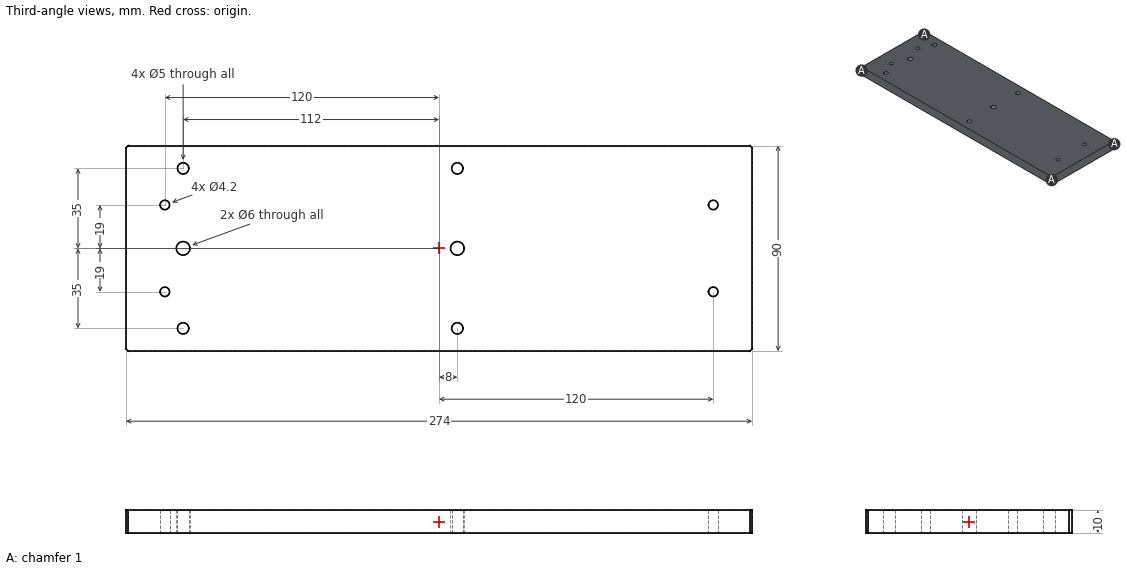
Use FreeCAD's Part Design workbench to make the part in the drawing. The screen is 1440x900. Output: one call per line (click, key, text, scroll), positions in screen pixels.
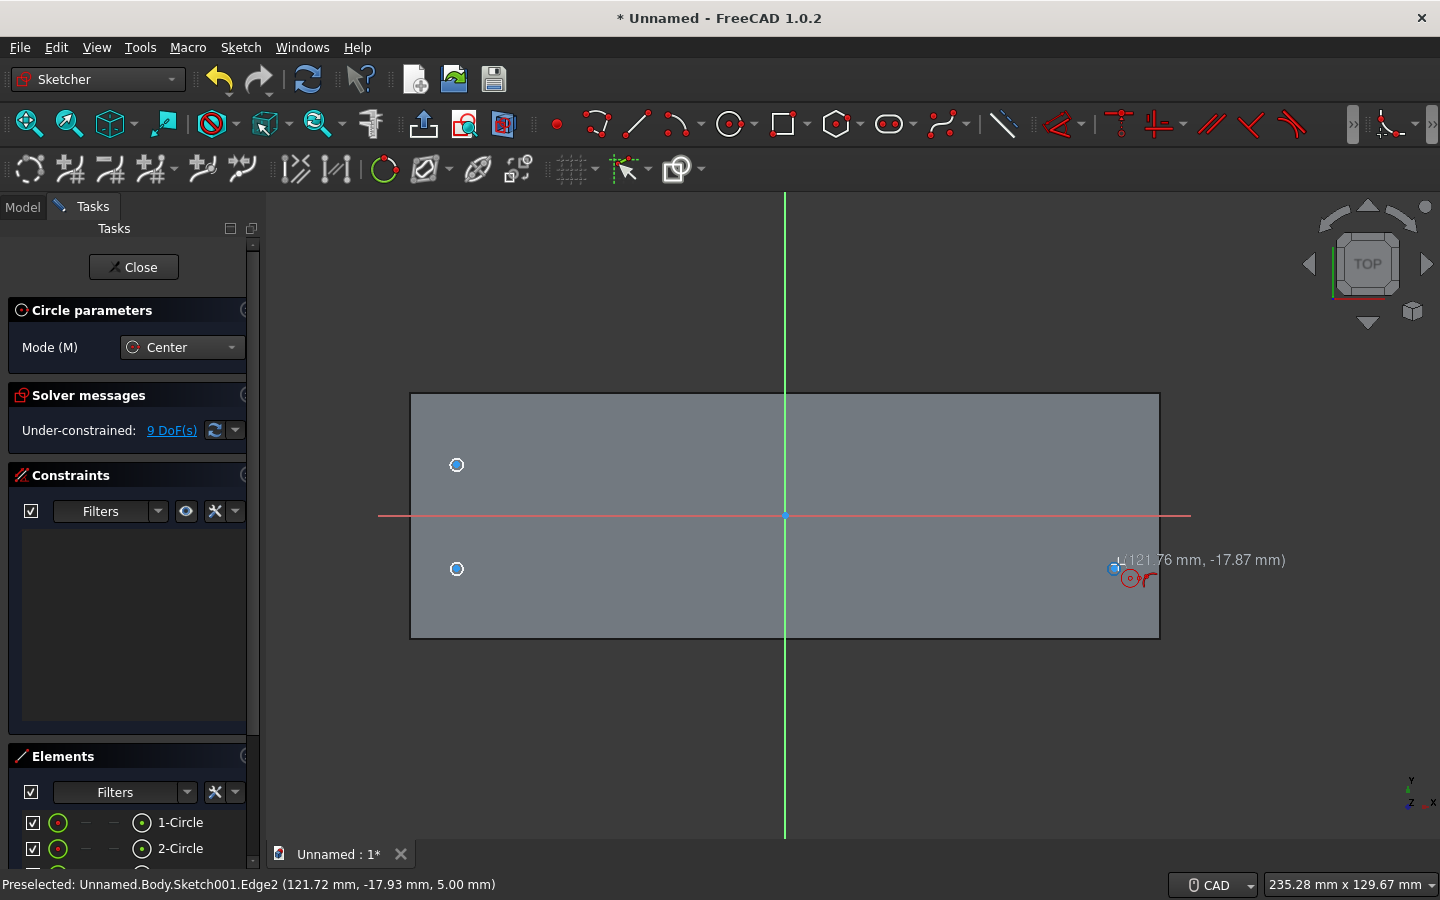
click(1114, 464)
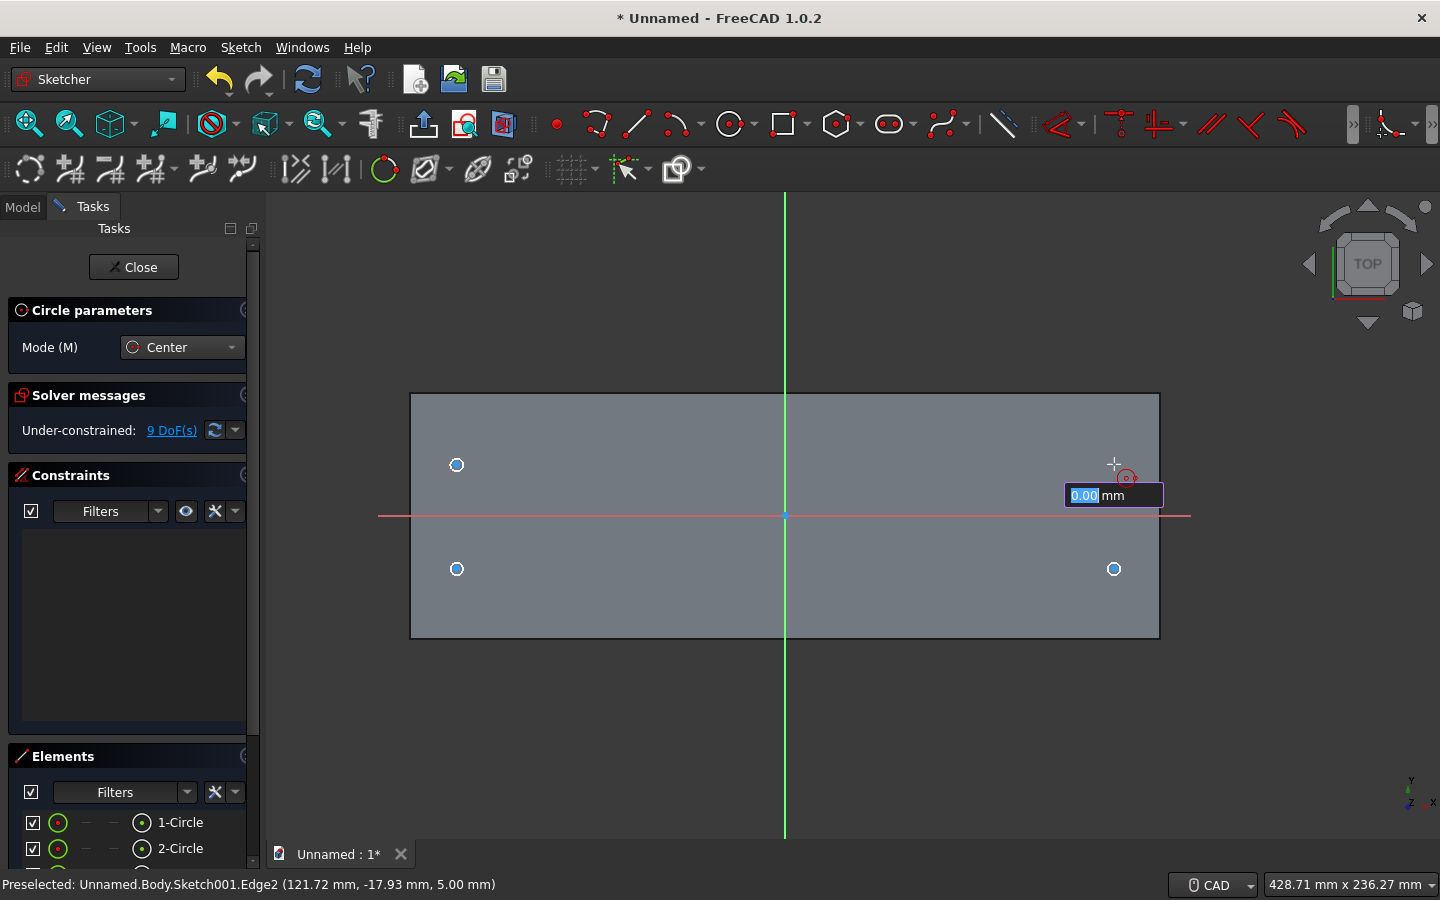
scroll(1118, 460, up, 6)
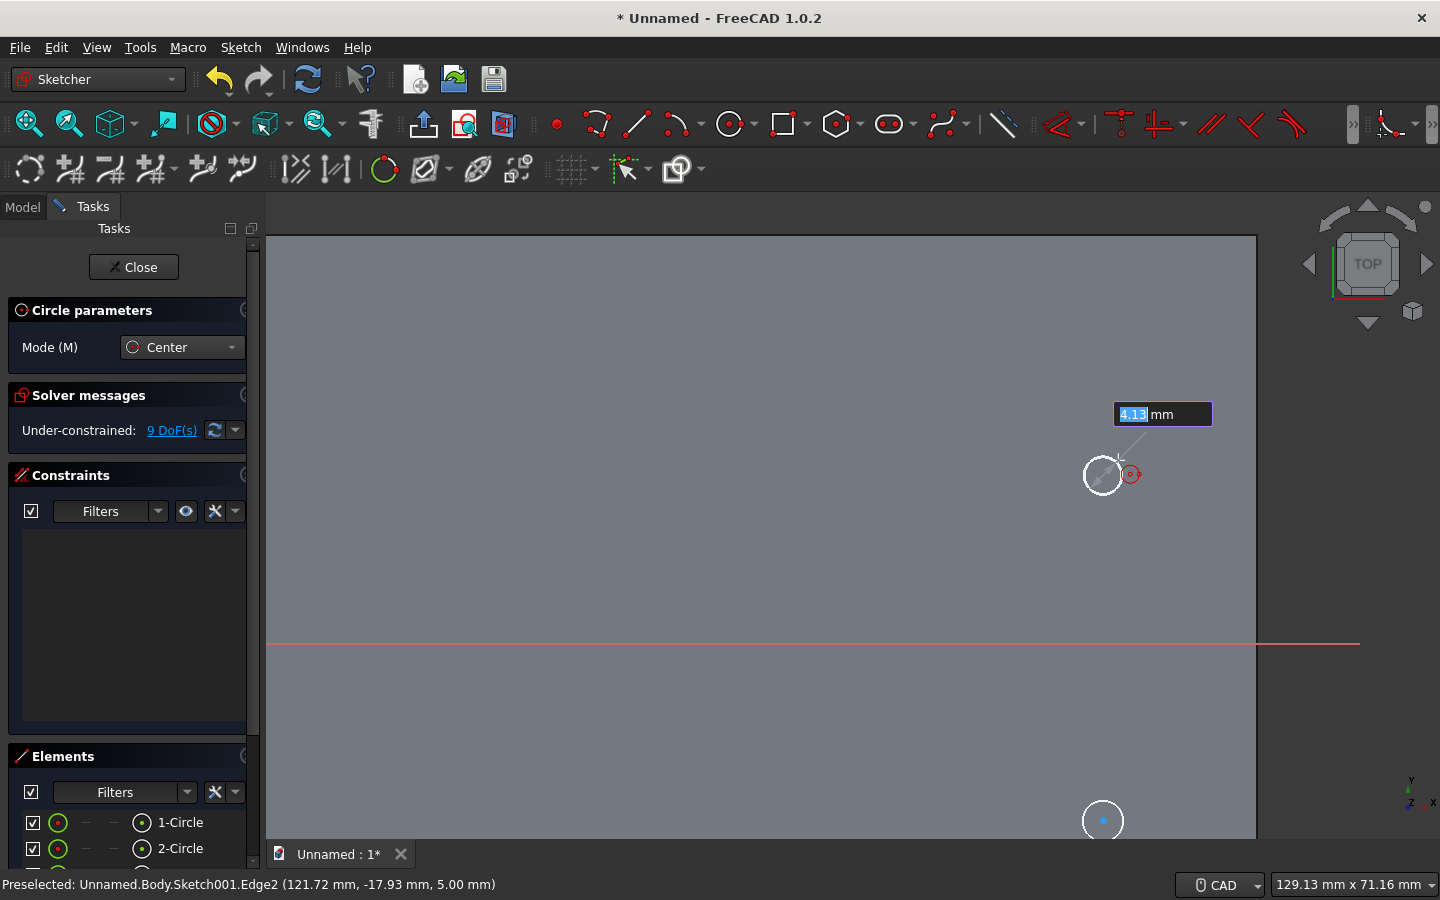
click(1115, 458)
key(Escape)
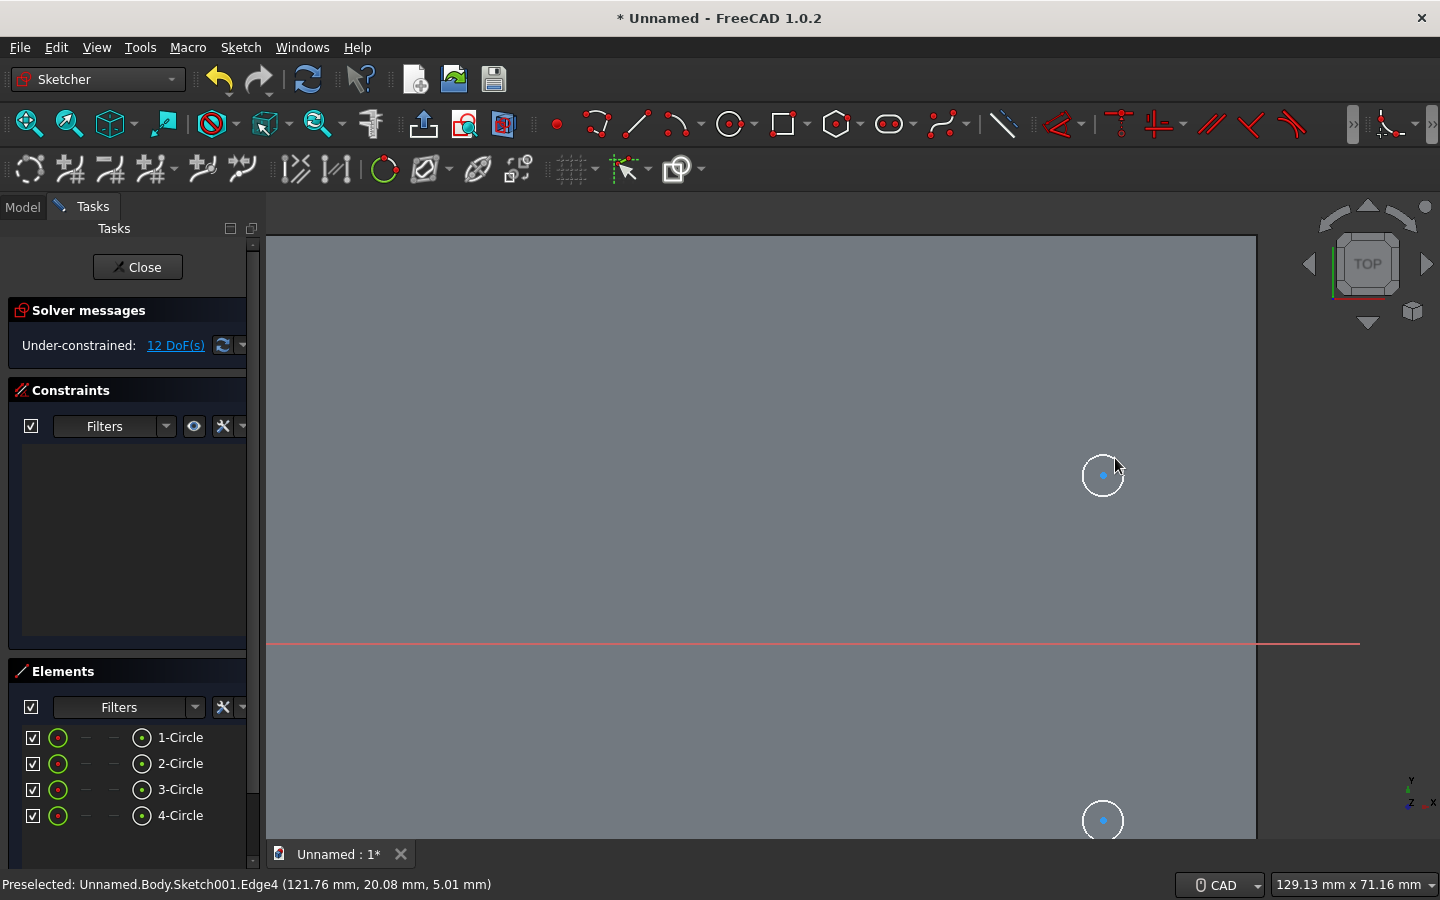
scroll(1118, 460, down, 6)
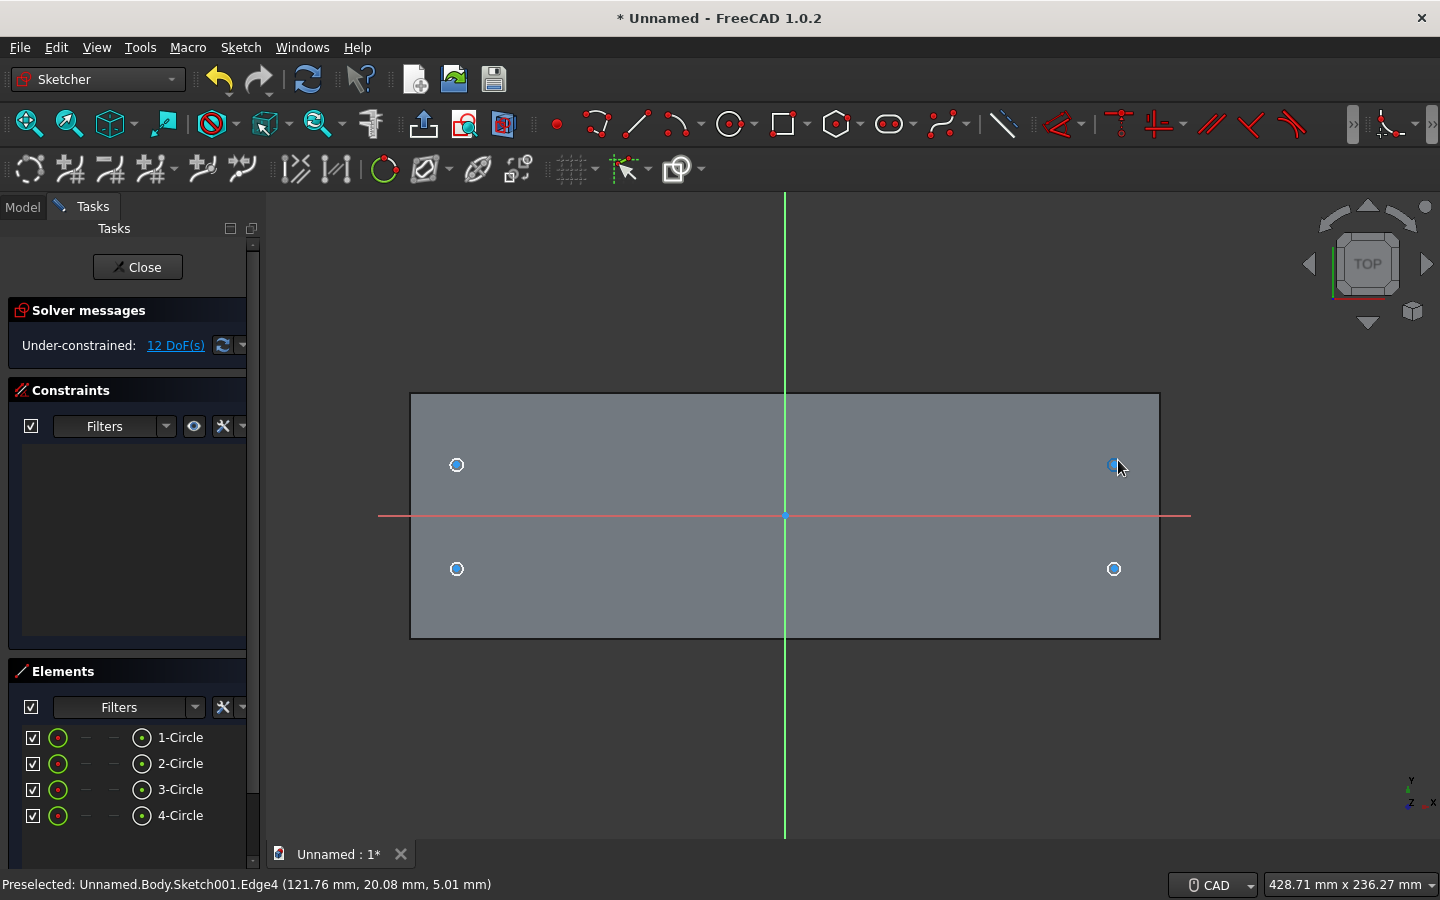
scroll(461, 461, up, 4)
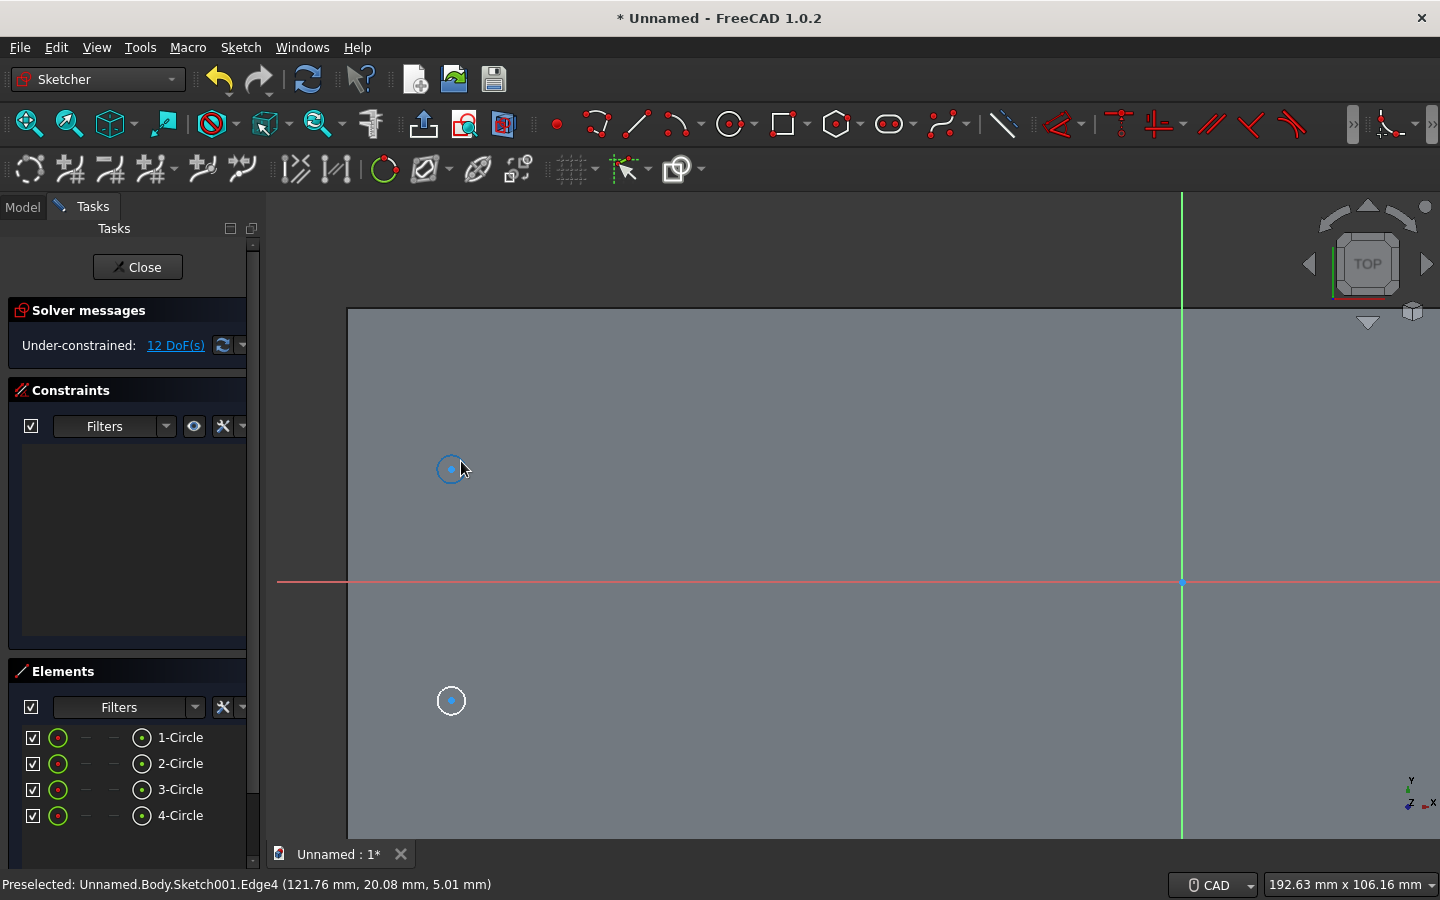
click(461, 459)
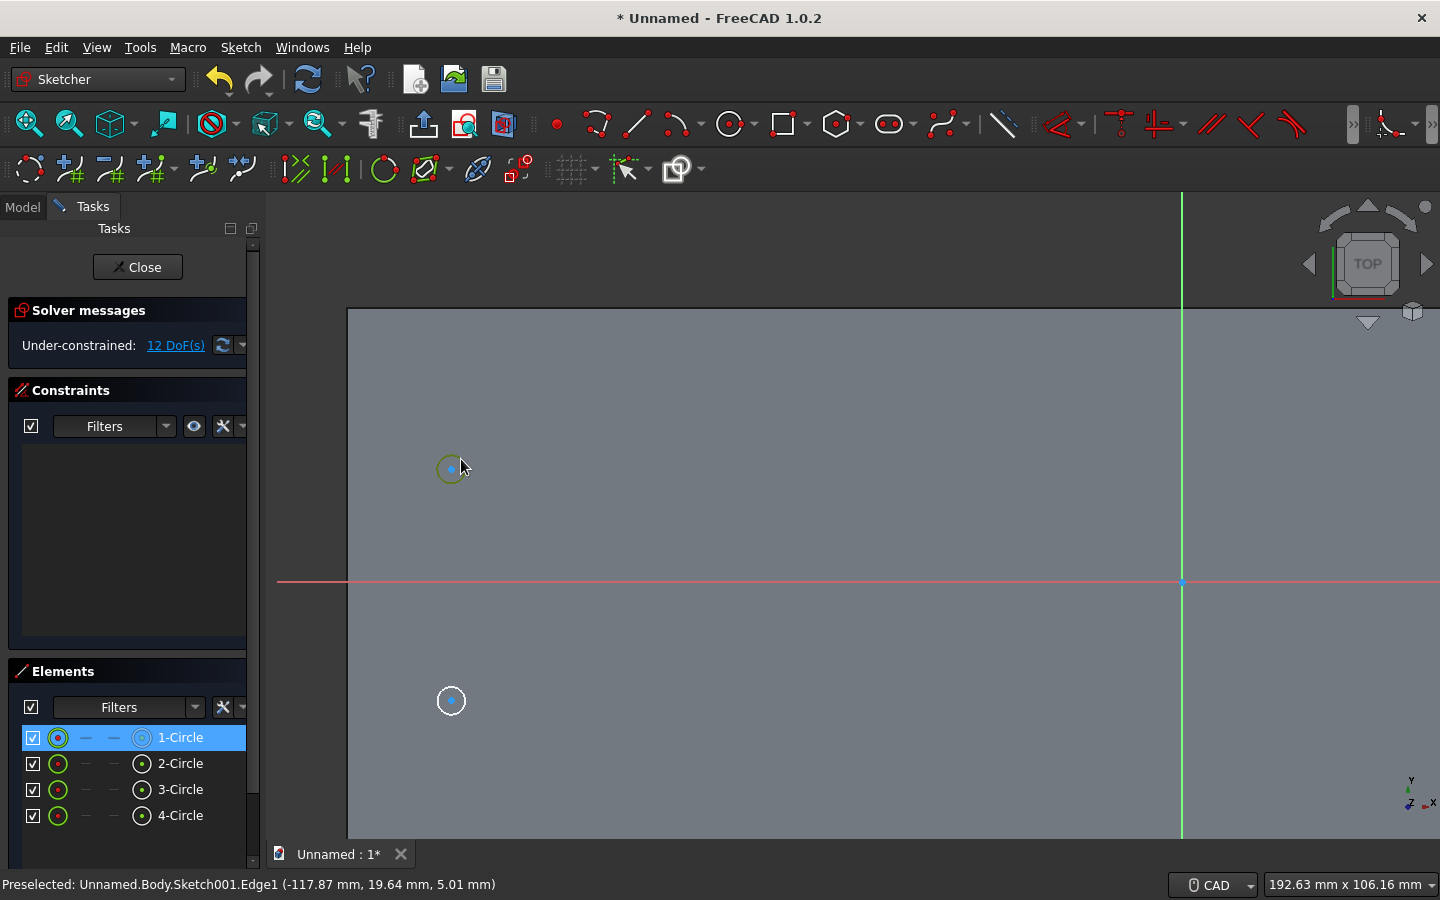
click(461, 691)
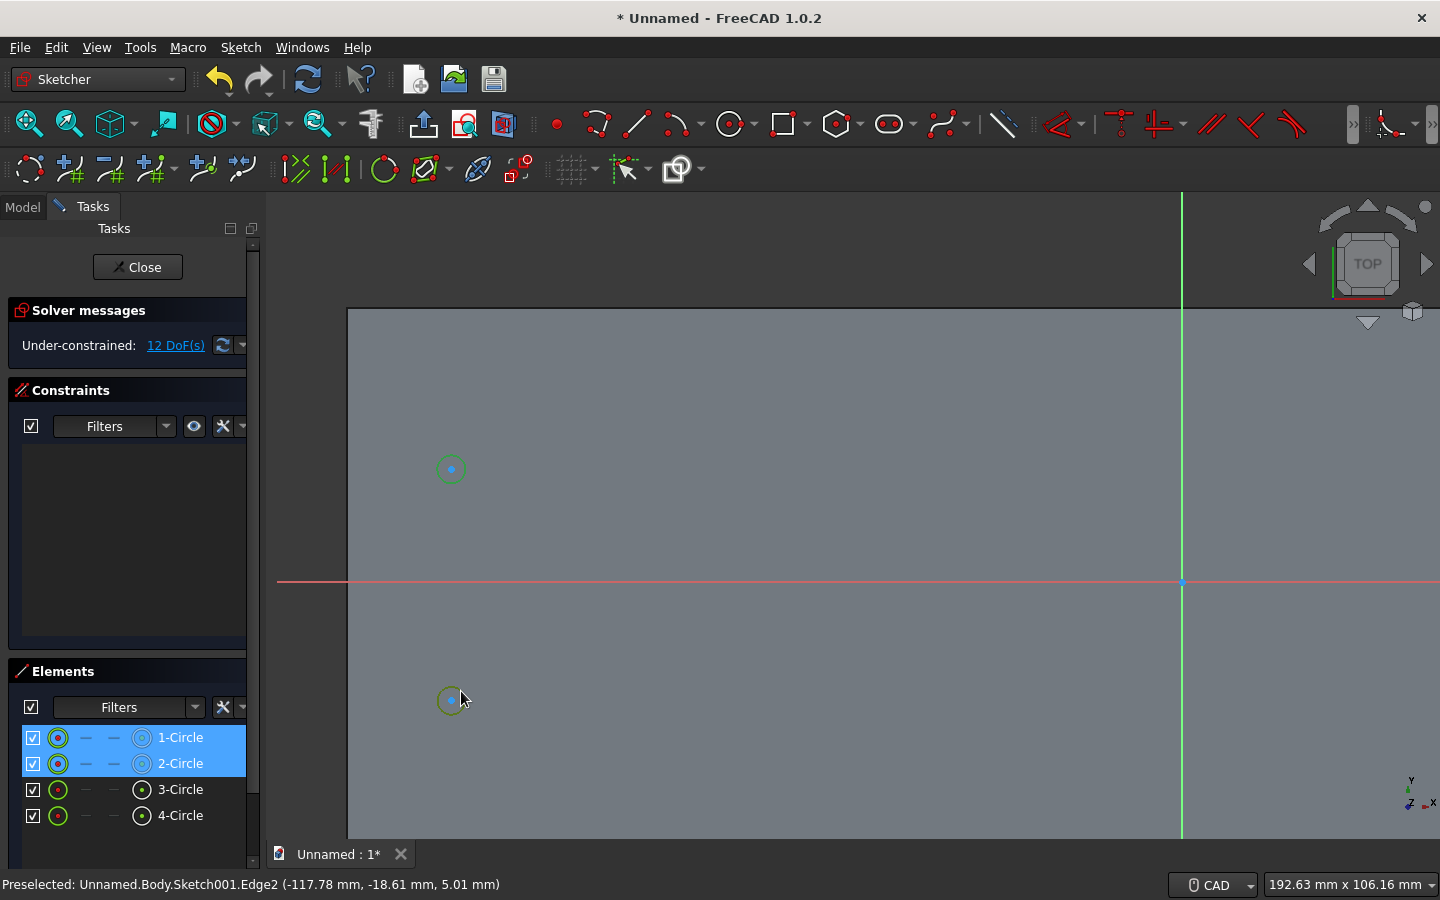
scroll(460, 461, down, 4)